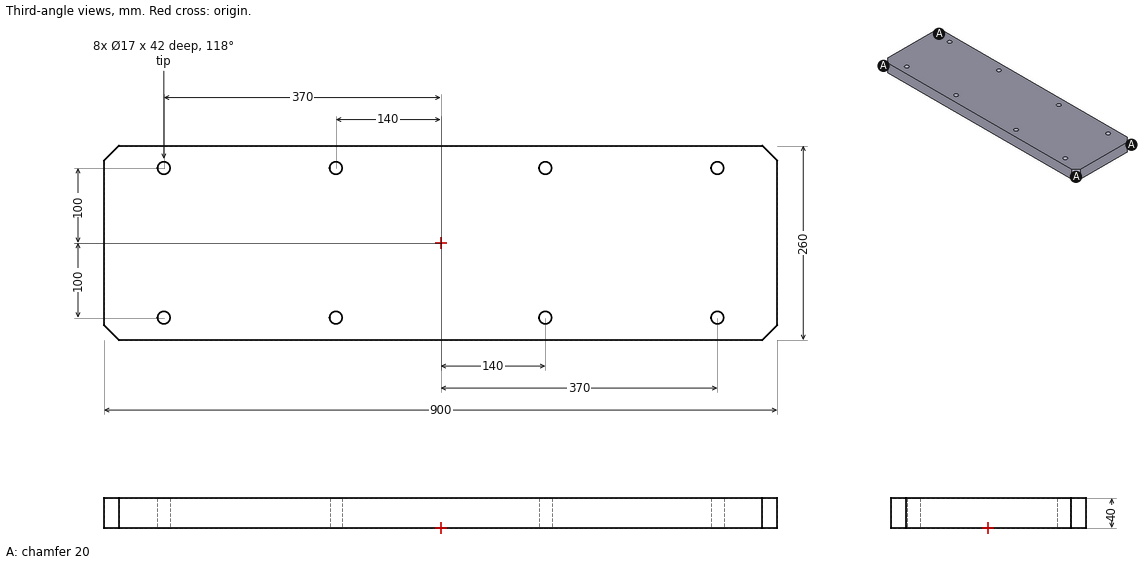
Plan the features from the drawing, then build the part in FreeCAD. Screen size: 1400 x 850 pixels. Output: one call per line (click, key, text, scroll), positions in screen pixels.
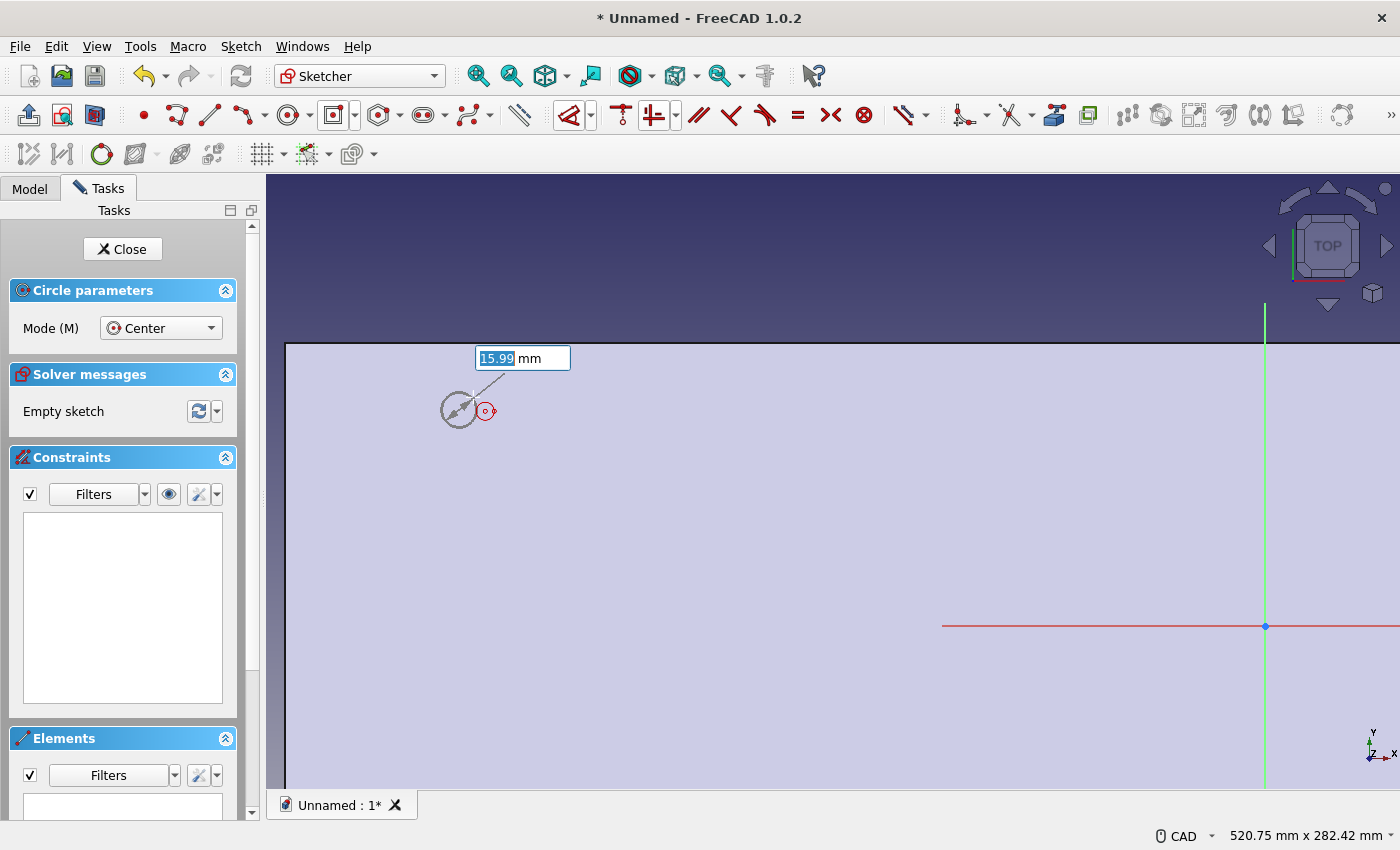
click(473, 395)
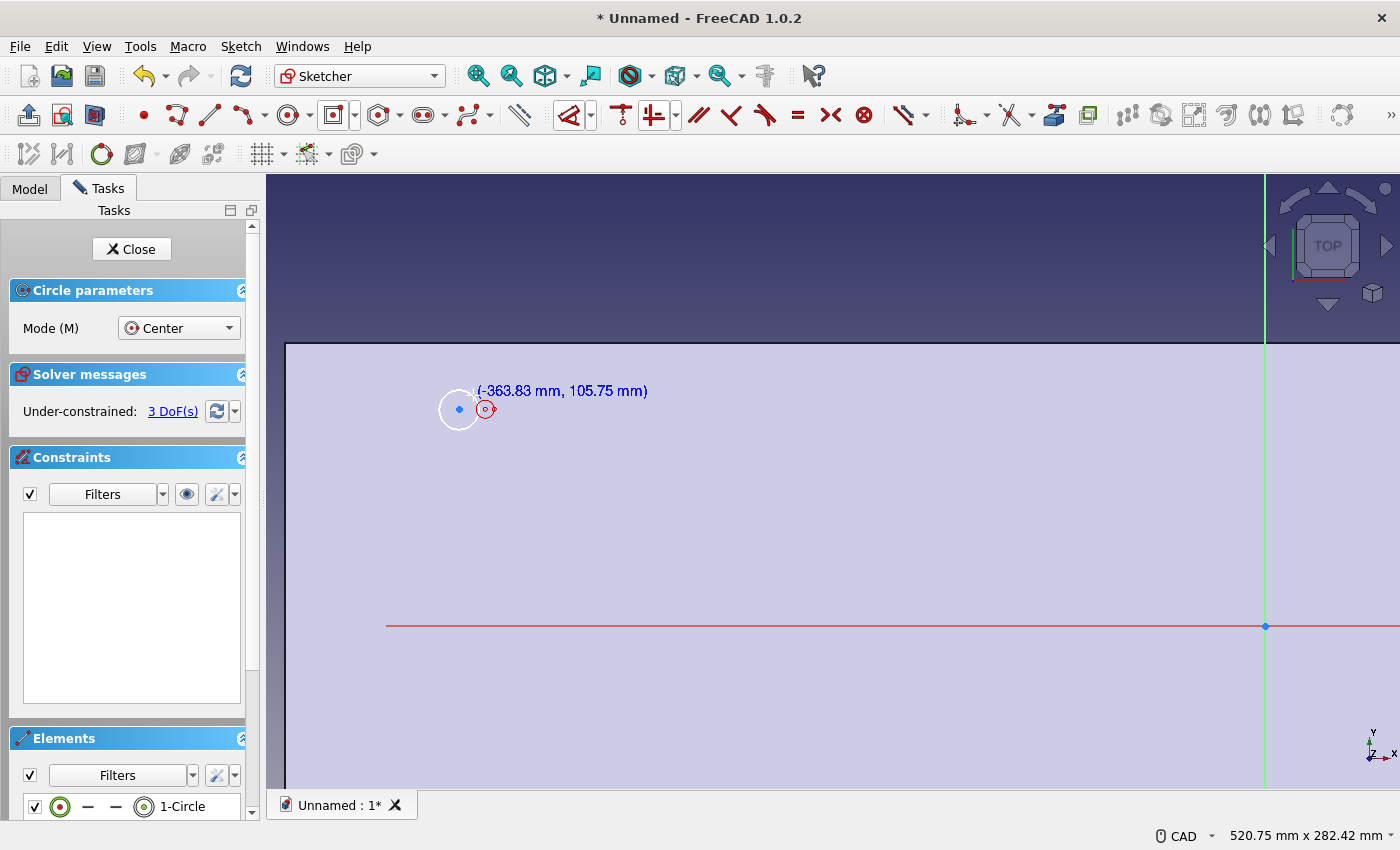
scroll(960, 409, up, 2)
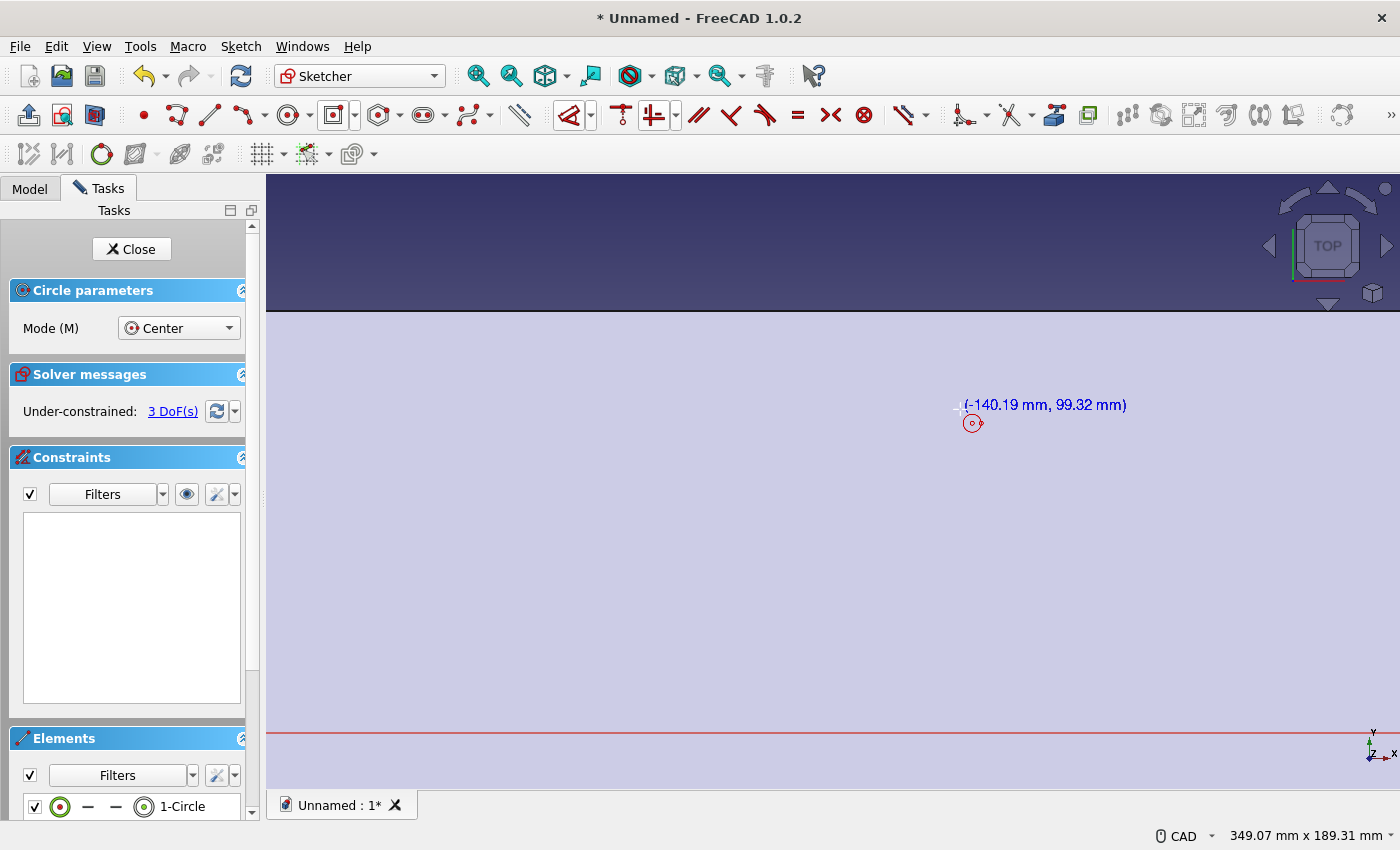
scroll(552, 399, down, 7)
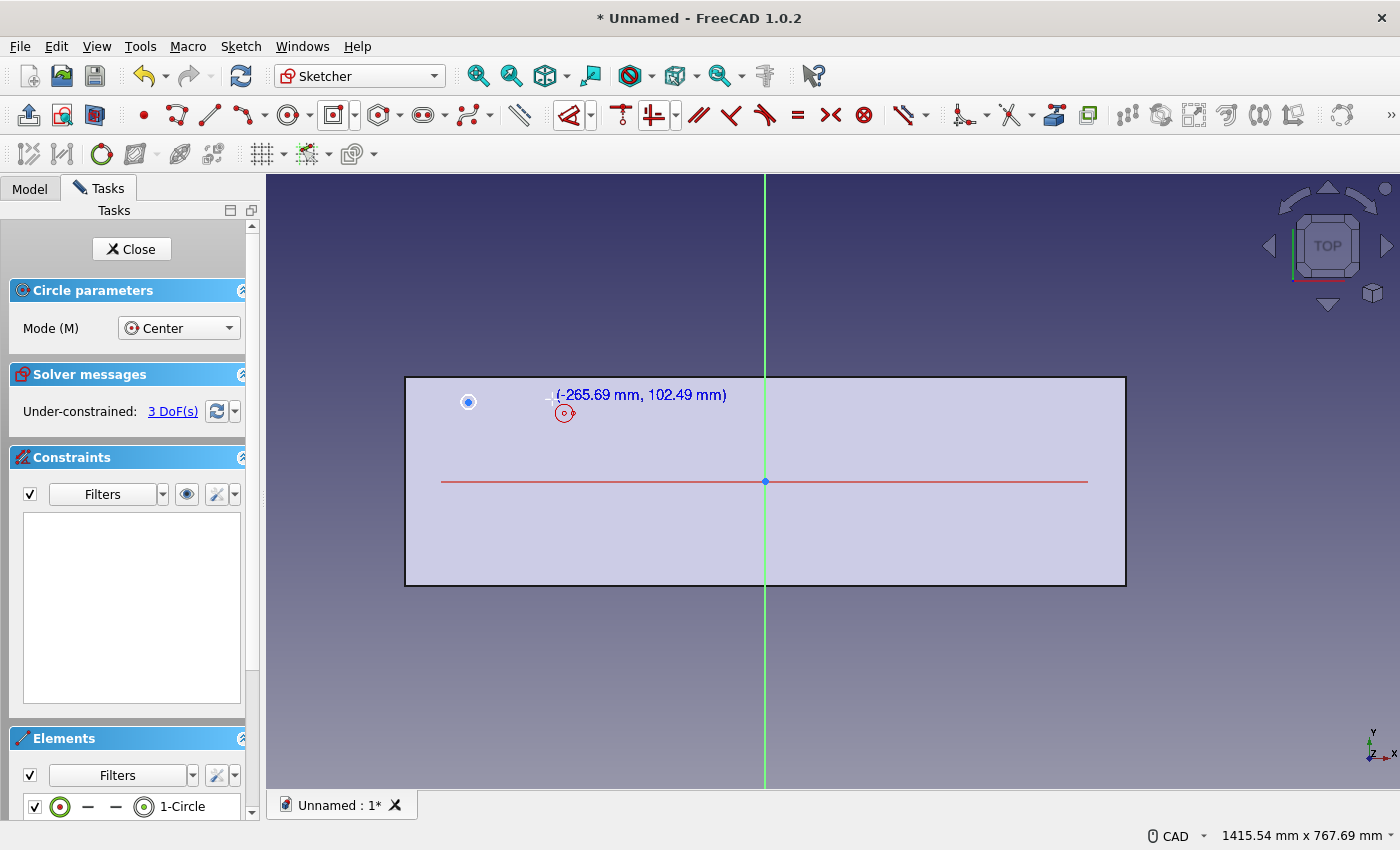
click(653, 402)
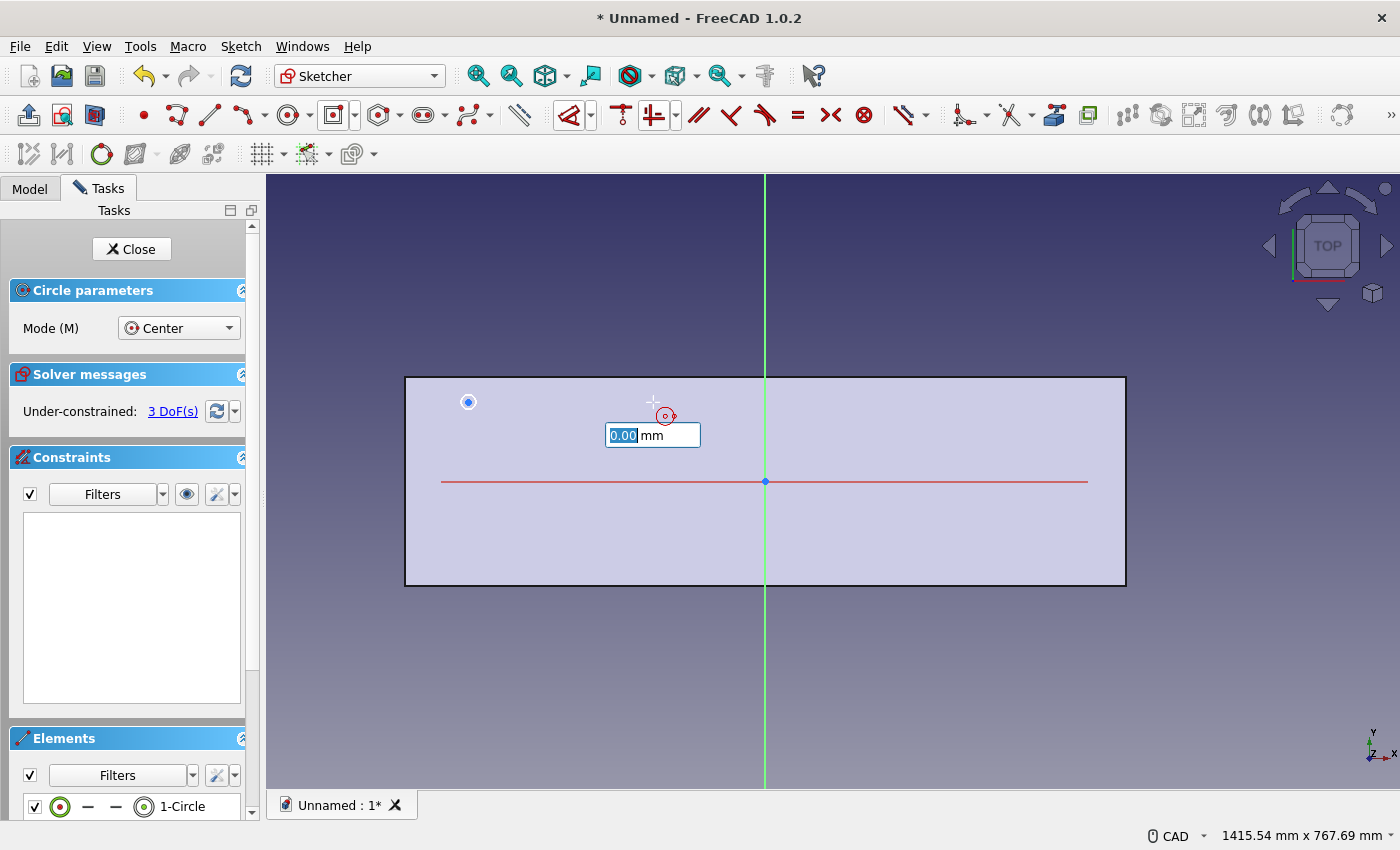
scroll(658, 397, up, 5)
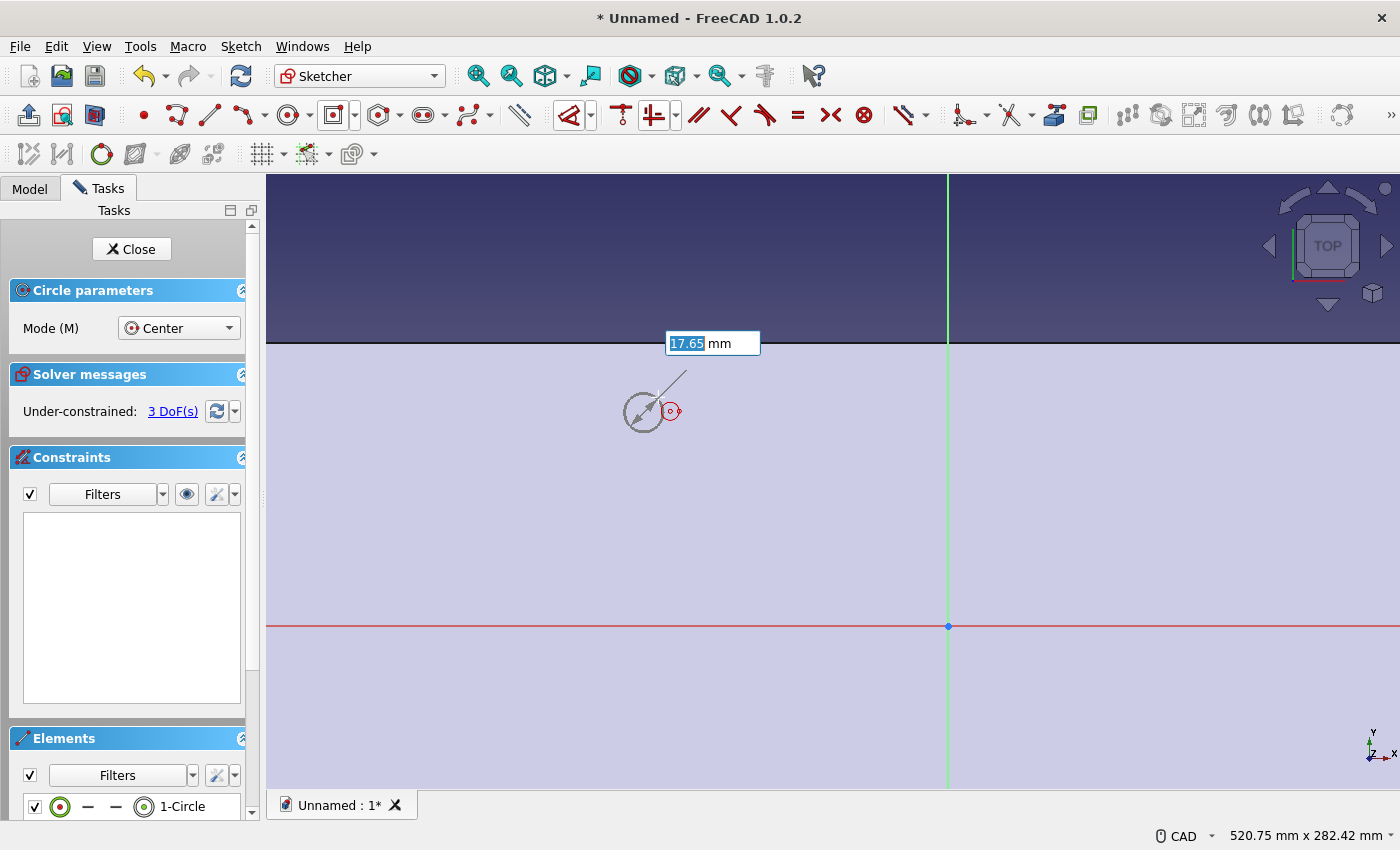
click(657, 396)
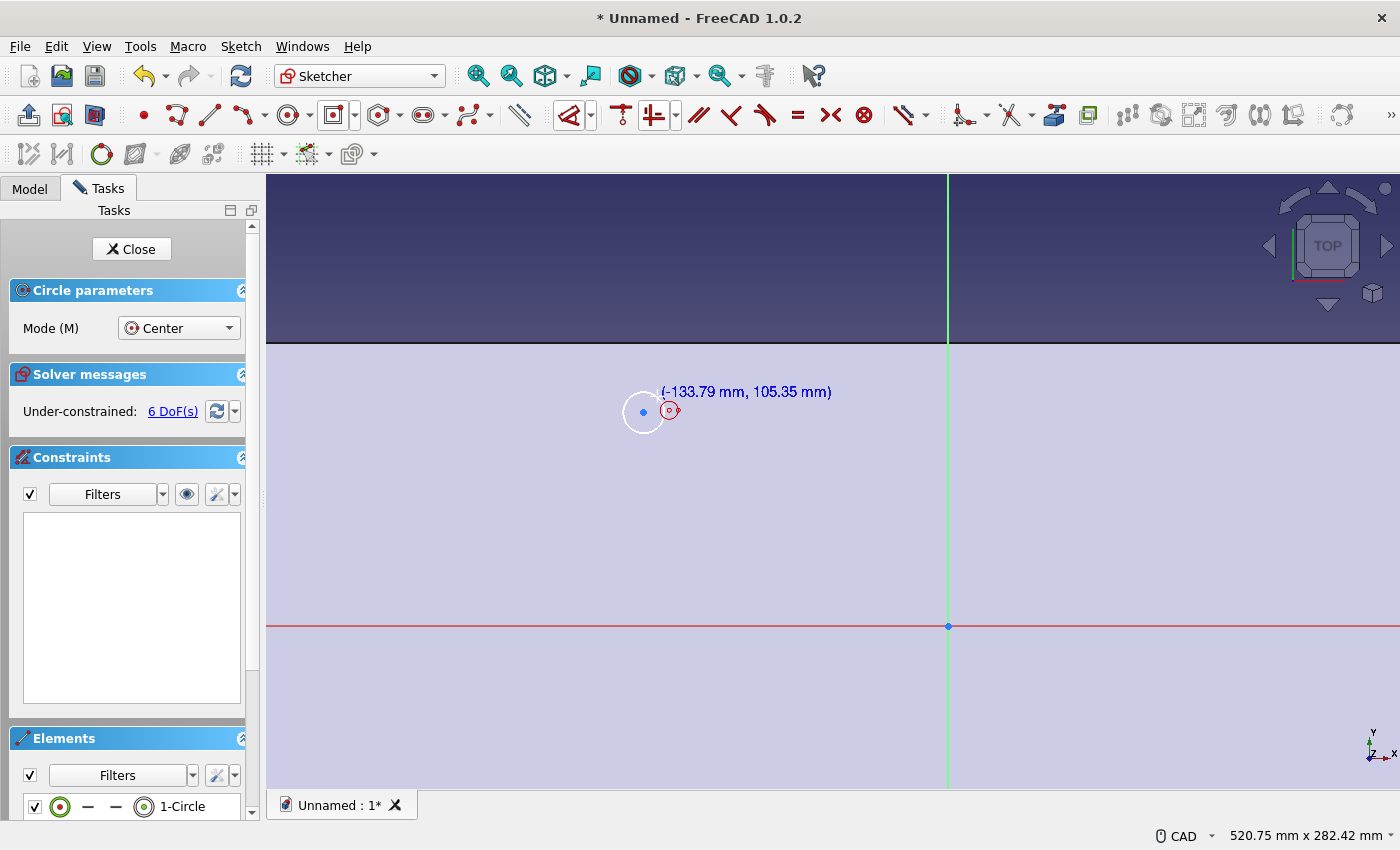
scroll(658, 397, down, 5)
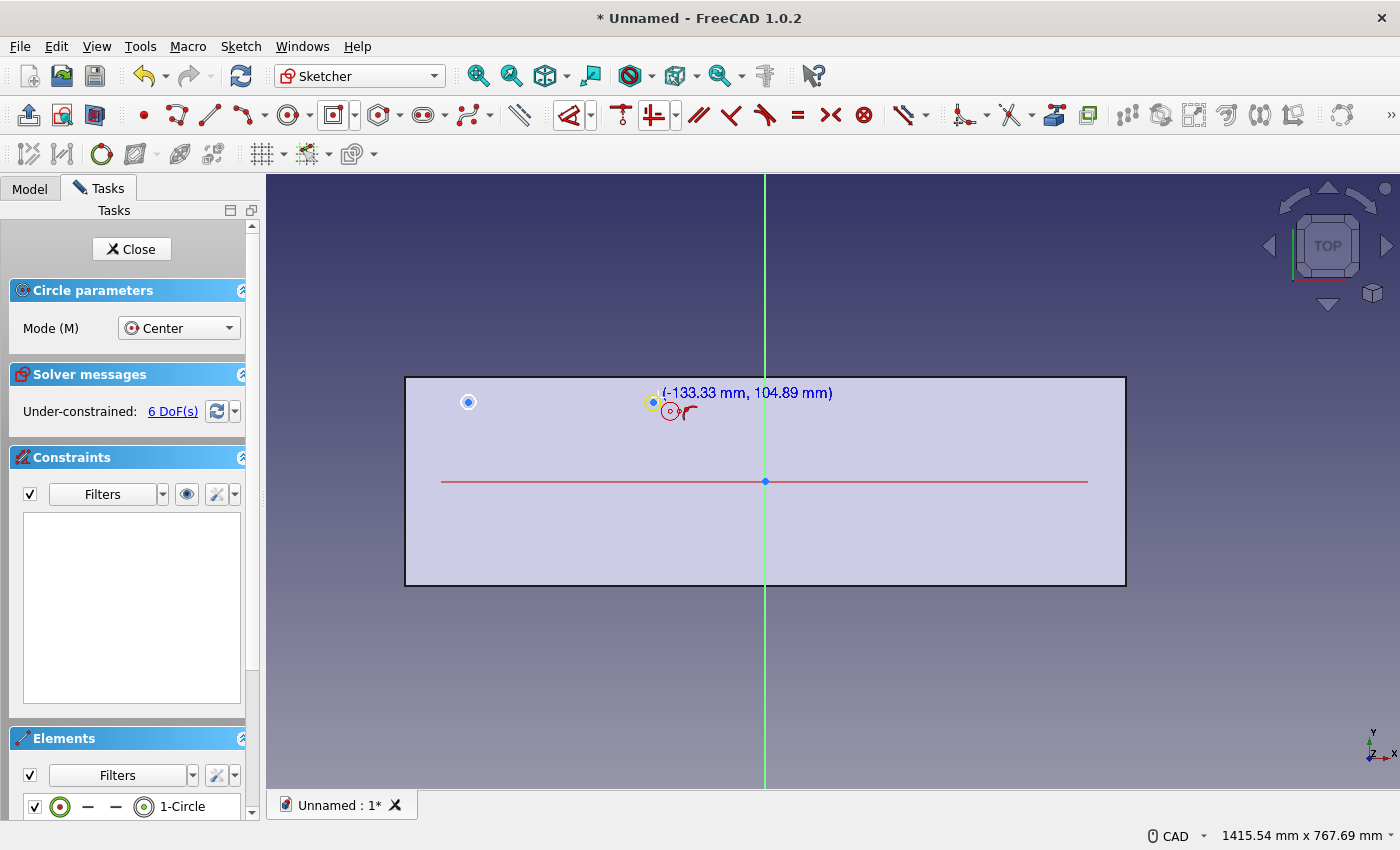
scroll(469, 562, up, 7)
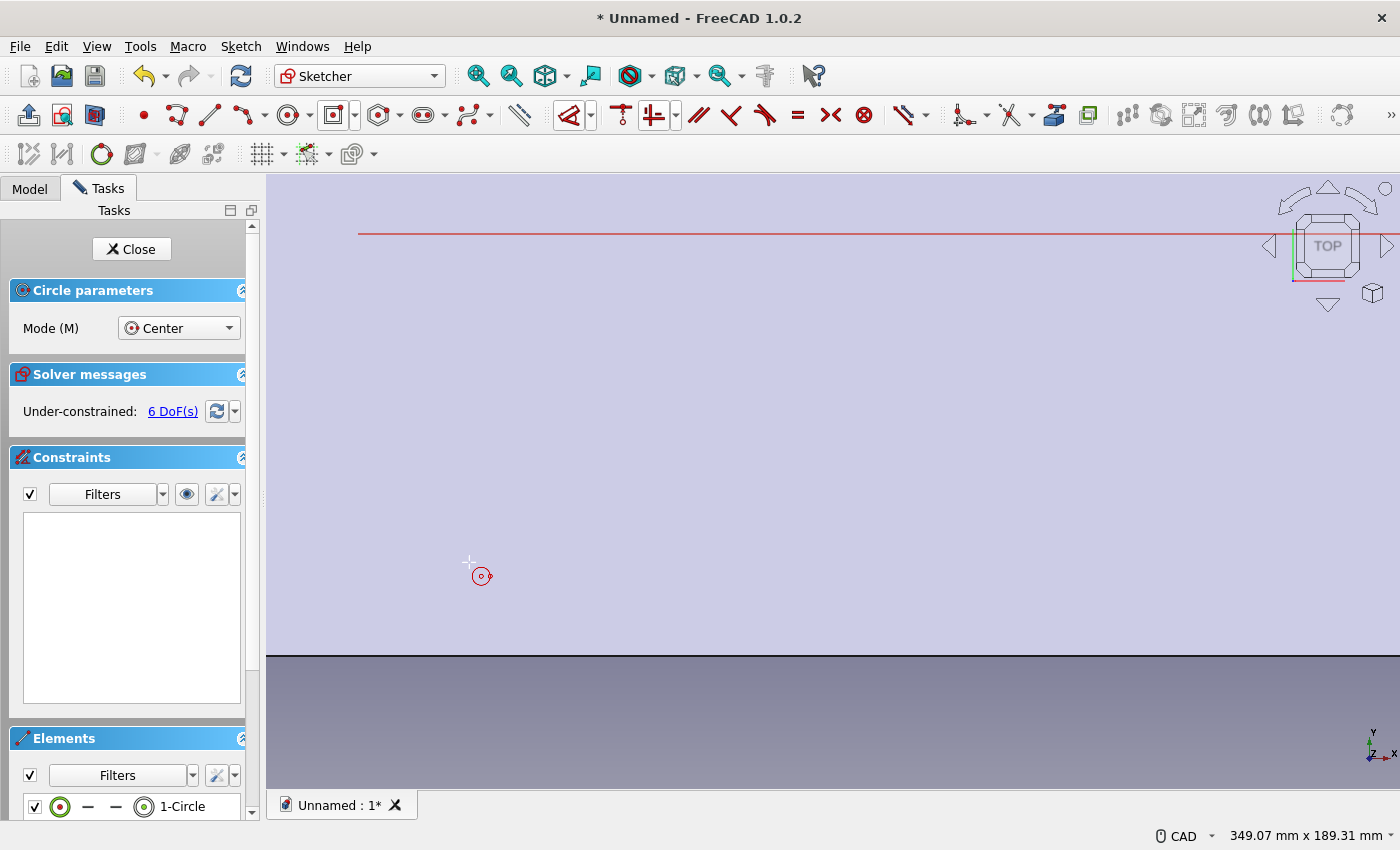
scroll(468, 562, down, 7)